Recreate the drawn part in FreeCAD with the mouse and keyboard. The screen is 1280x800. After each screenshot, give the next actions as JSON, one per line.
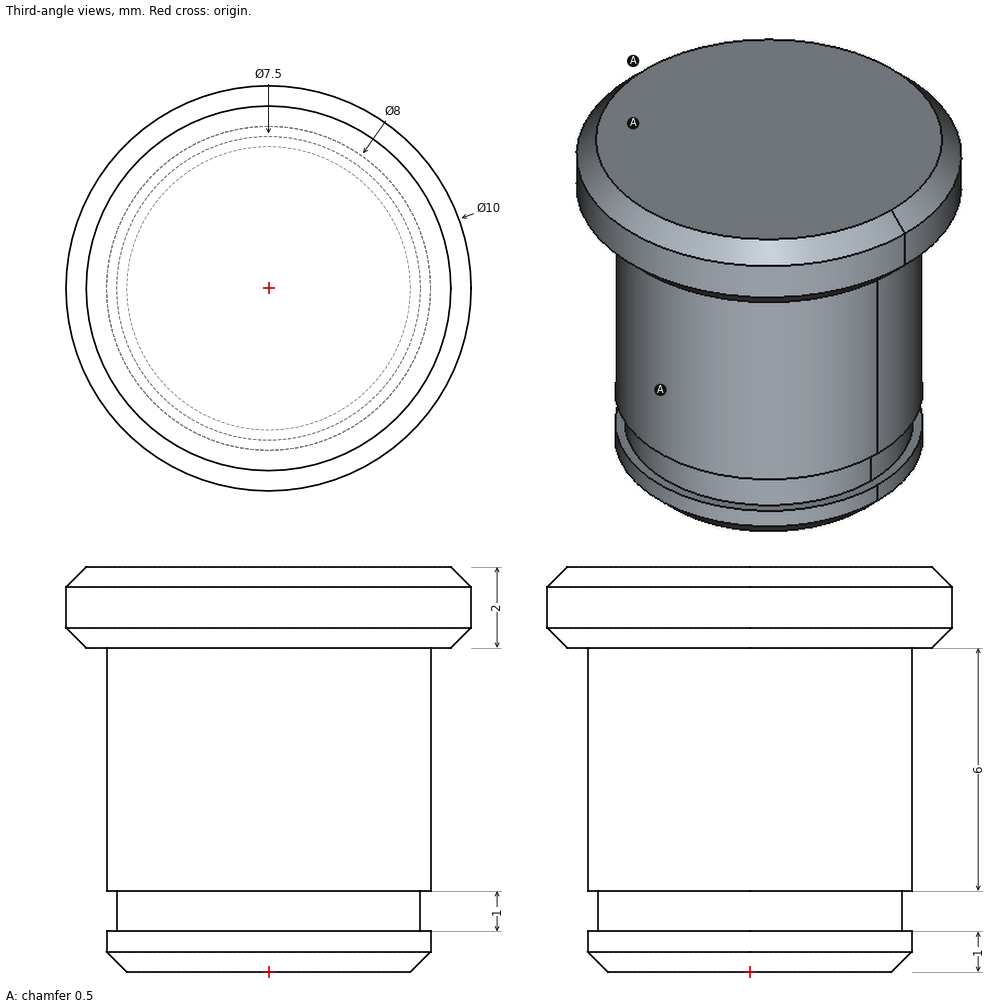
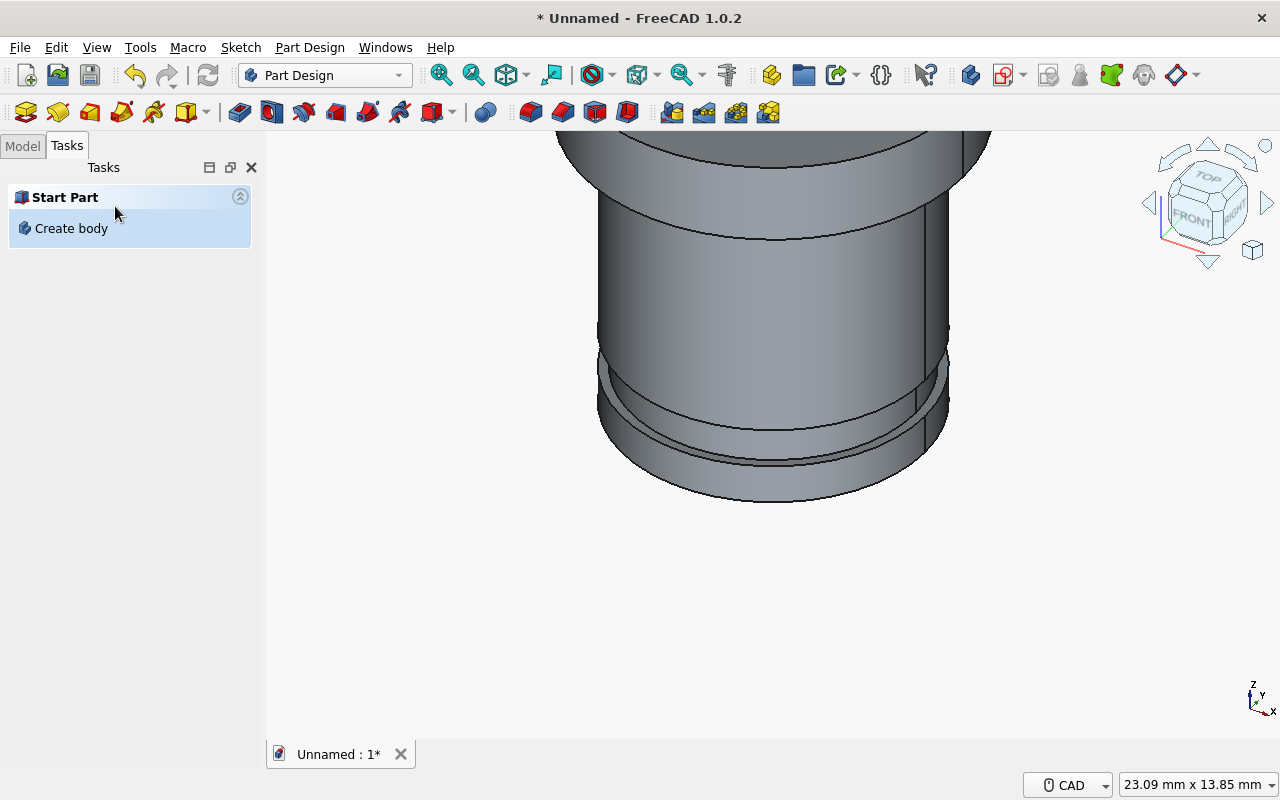
{"action": "left_click", "coordinate": [442, 76]}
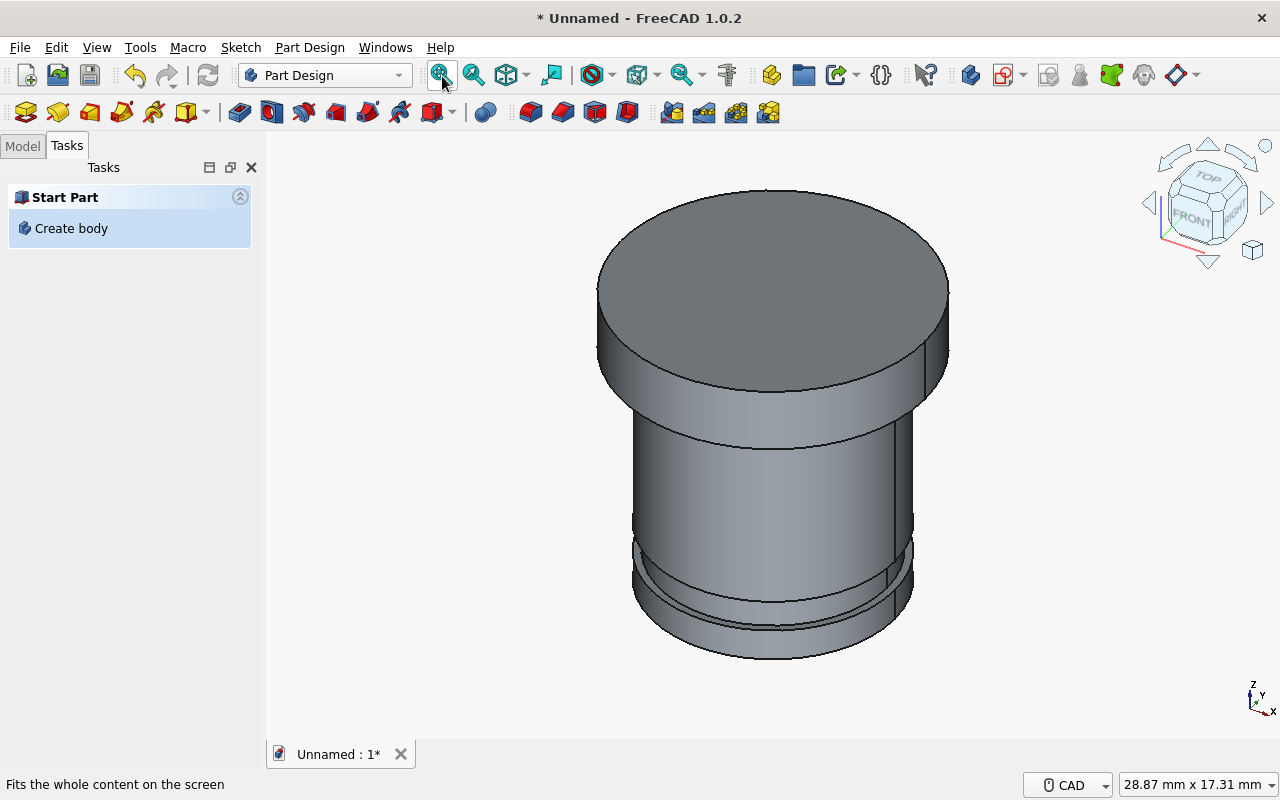
{"action": "left_click", "coordinate": [598, 301]}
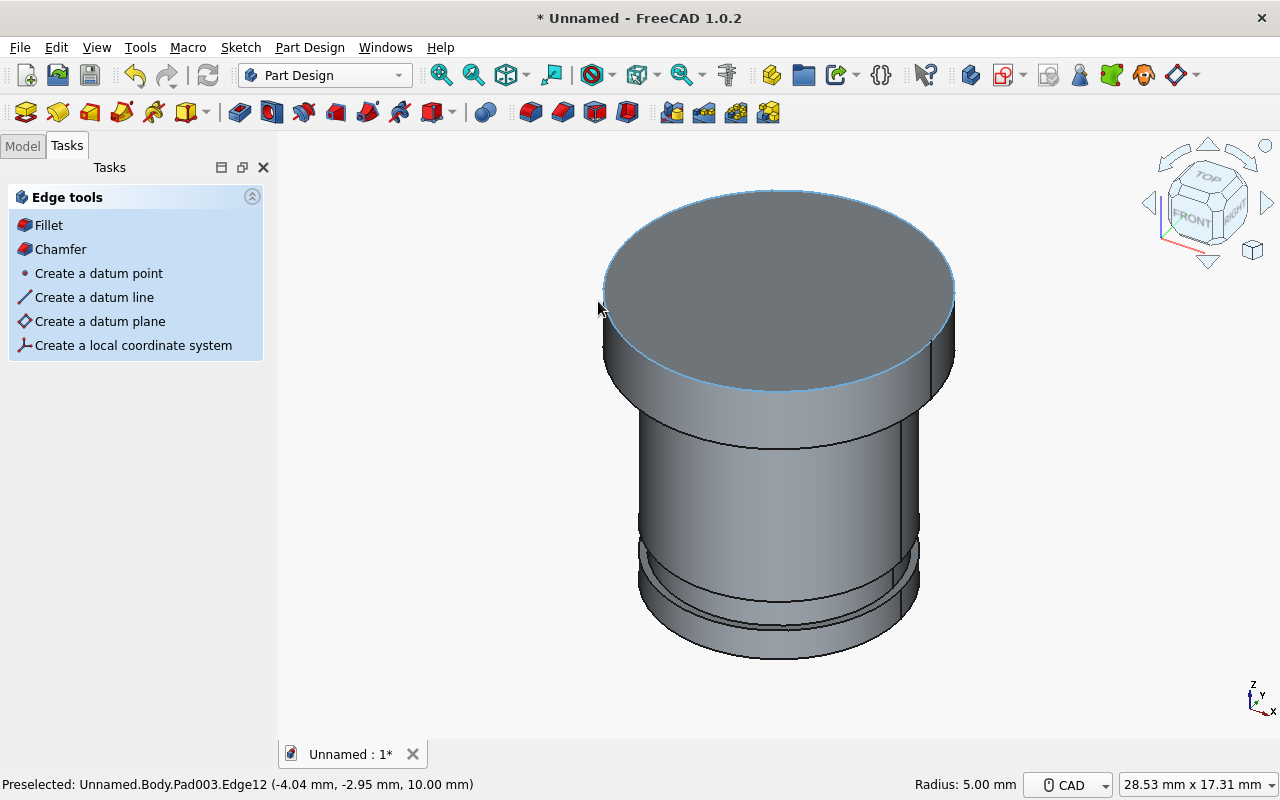
{"action": "key", "text": "0"}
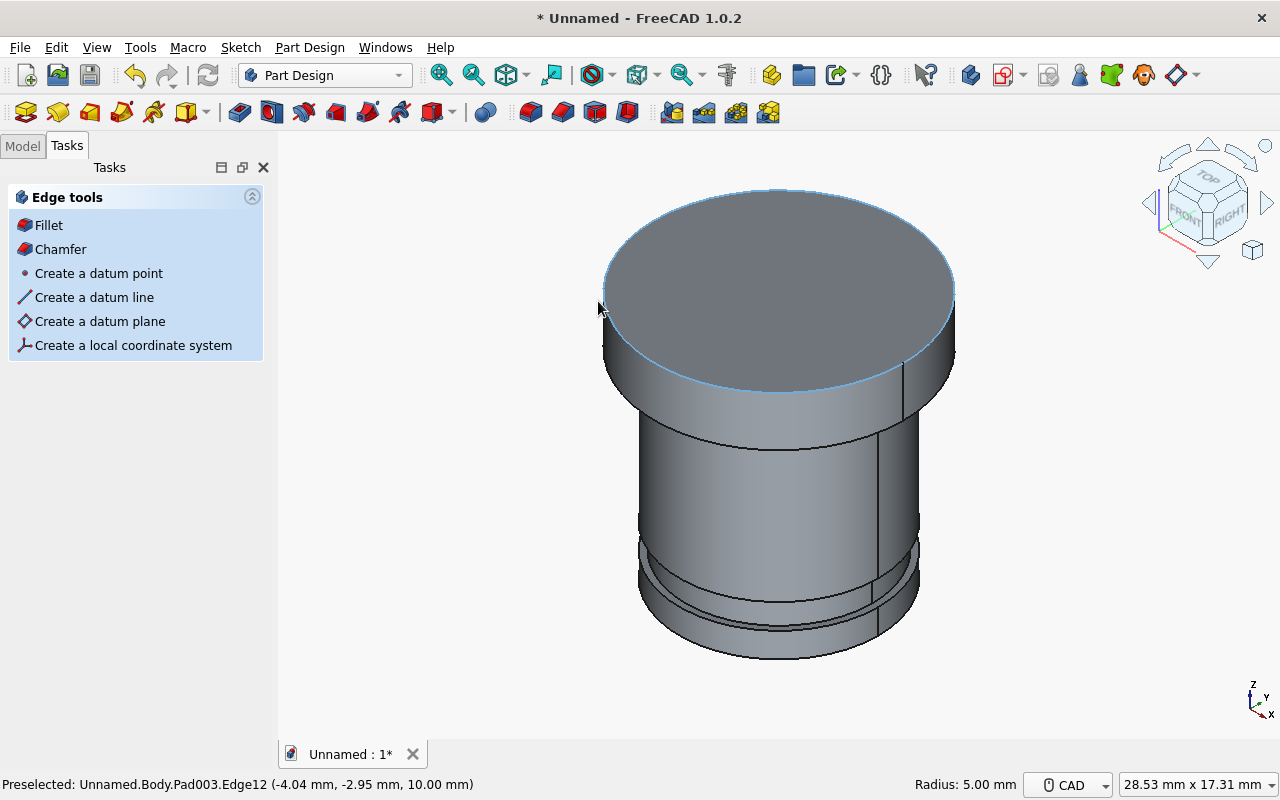
{"action": "key", "text": "2"}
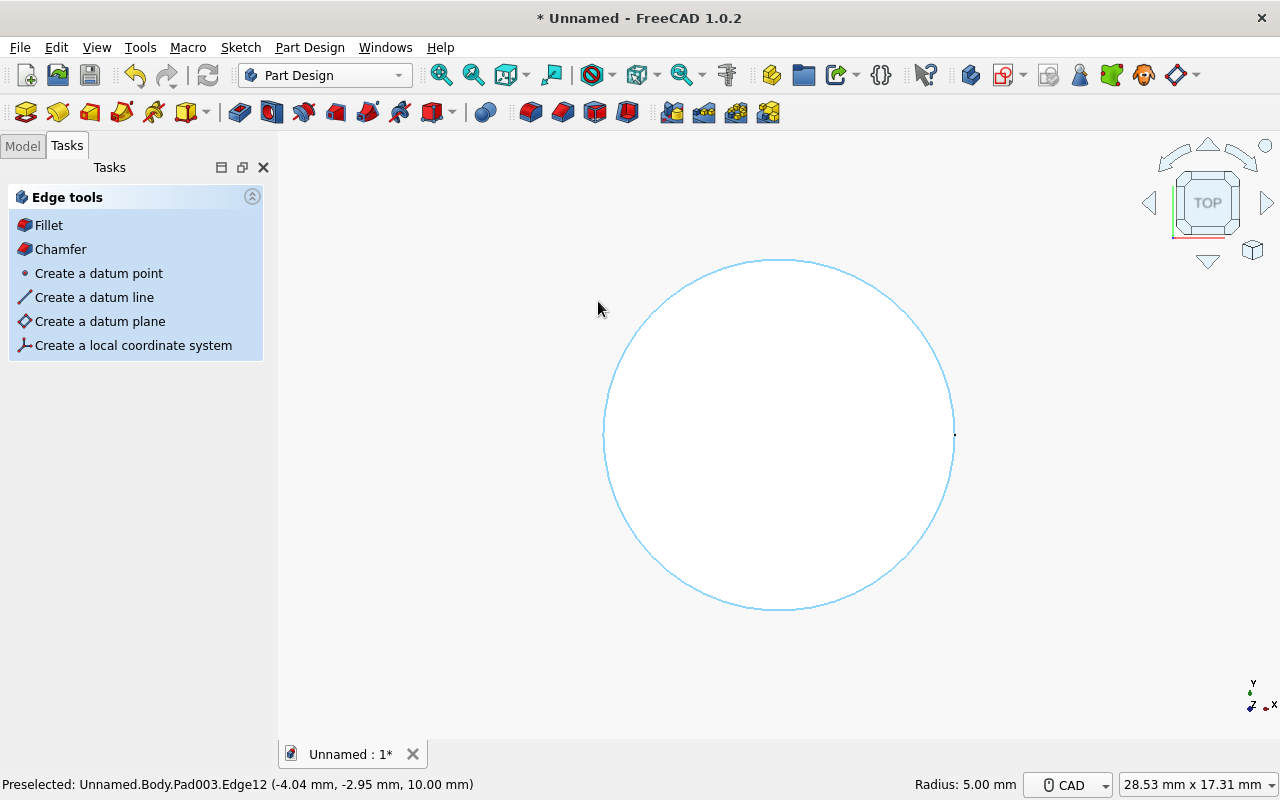
{"action": "key", "text": "1"}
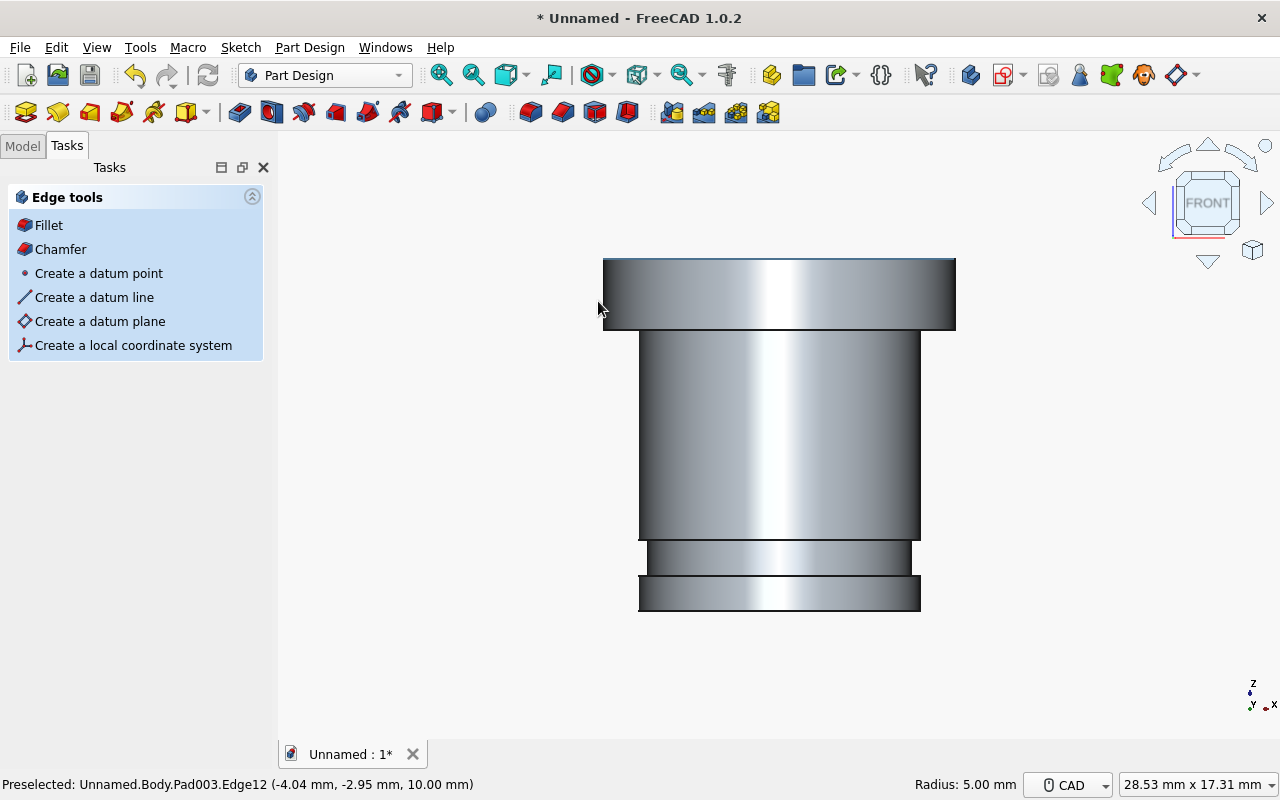
{"action": "left_click", "coordinate": [637, 329], "text": "ctrl"}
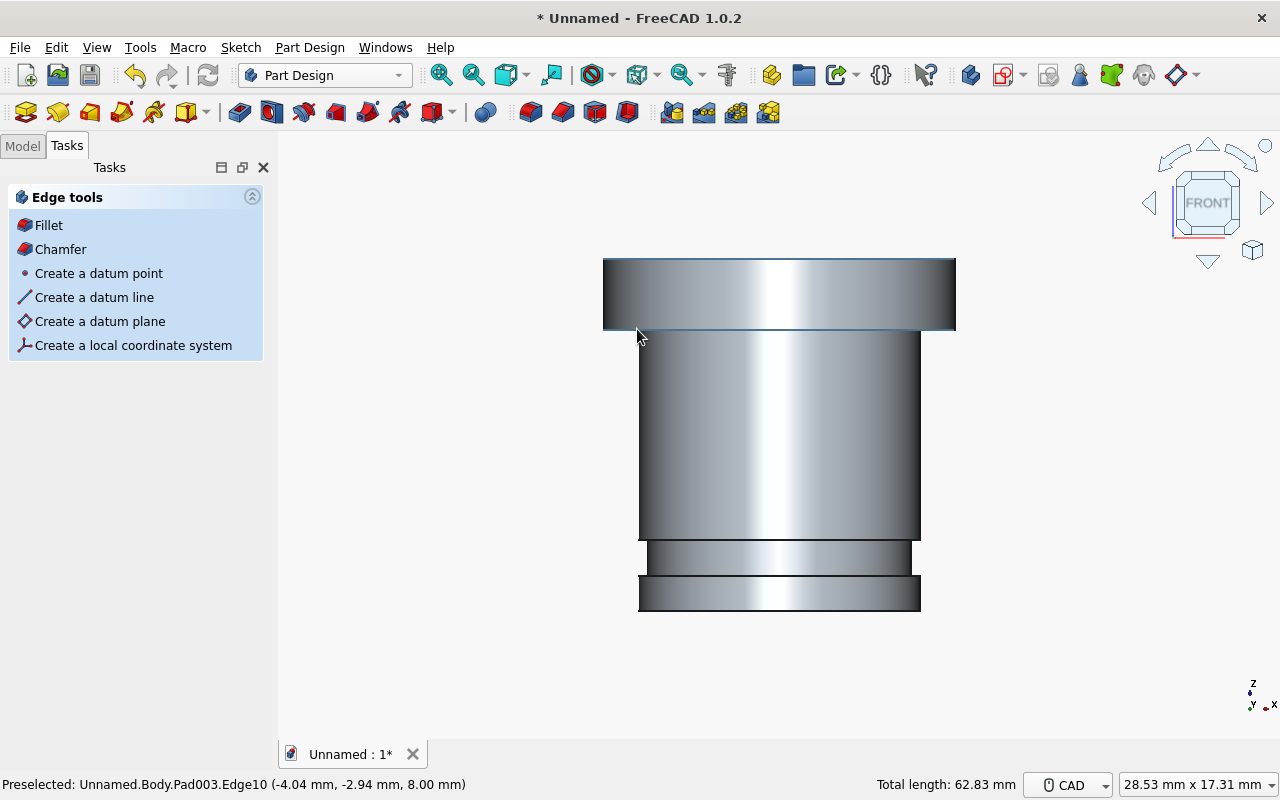
{"action": "left_click", "coordinate": [665, 610], "text": "ctrl"}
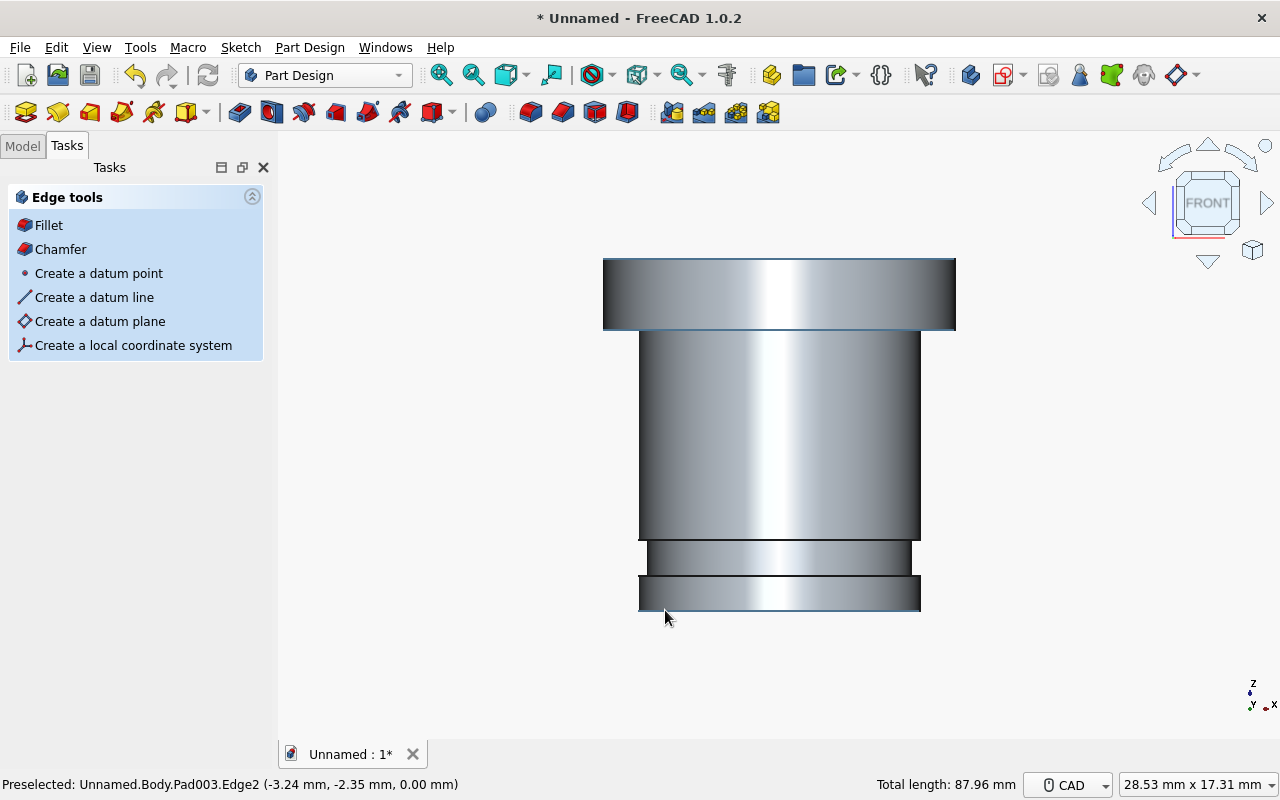
{"action": "left_click", "coordinate": [564, 112]}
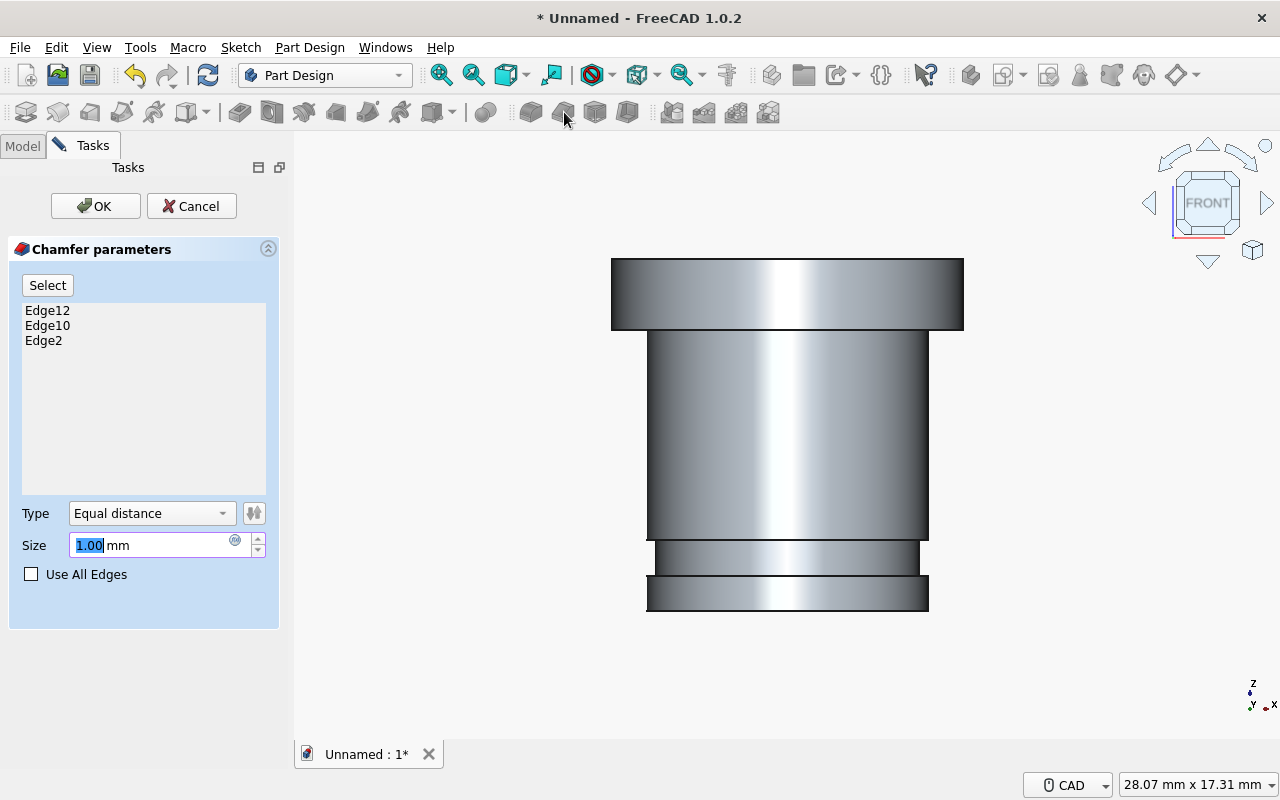
{"action": "type", "text": "0.5"}
{"action": "key", "text": "Tab"}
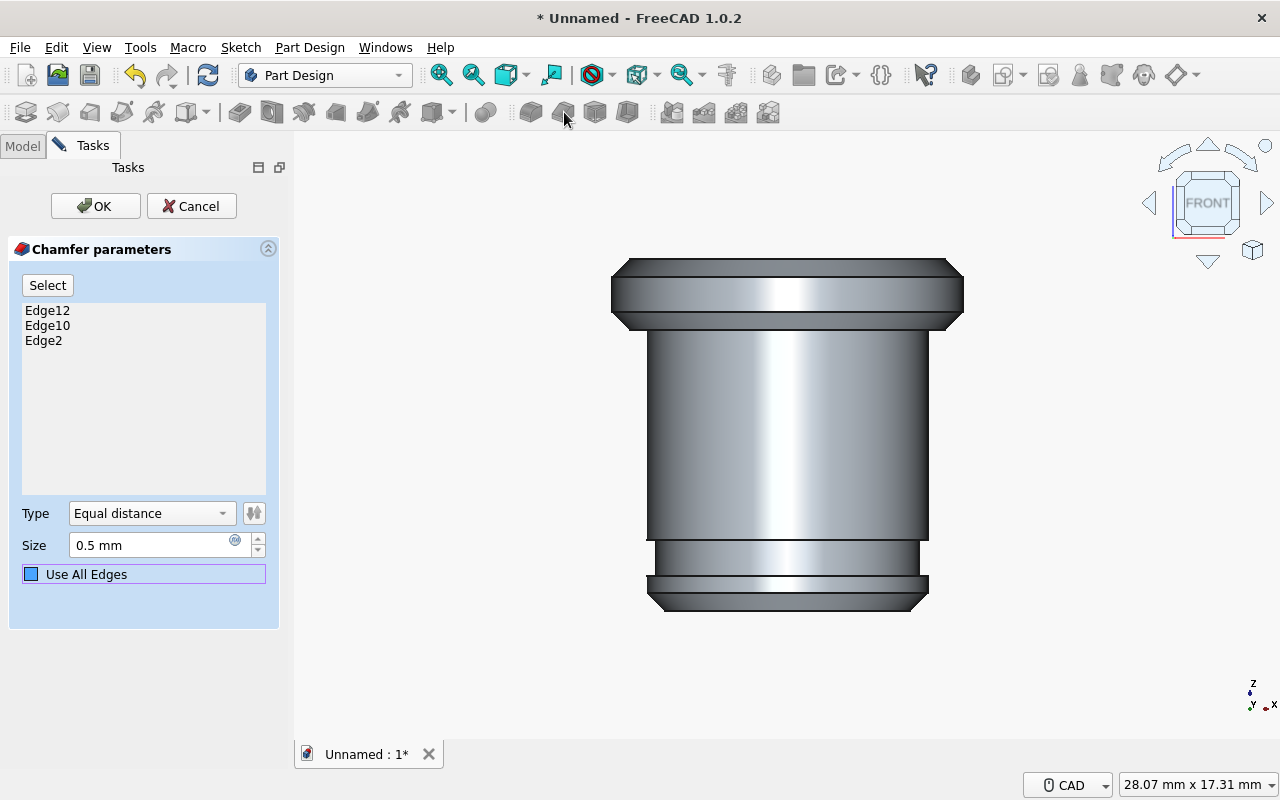
{"action": "left_click", "coordinate": [96, 206]}